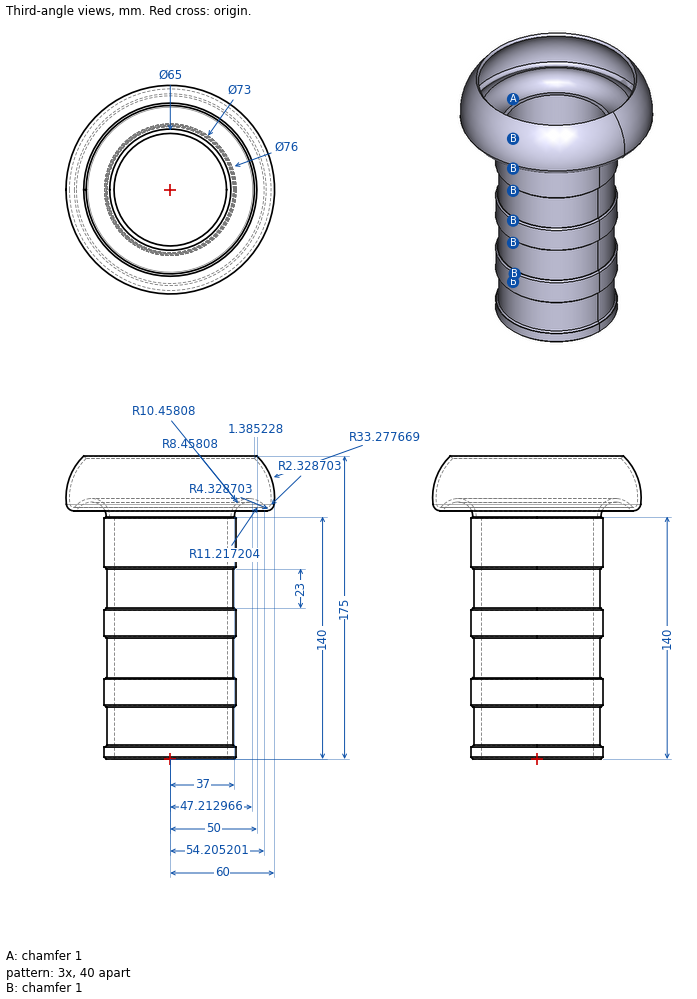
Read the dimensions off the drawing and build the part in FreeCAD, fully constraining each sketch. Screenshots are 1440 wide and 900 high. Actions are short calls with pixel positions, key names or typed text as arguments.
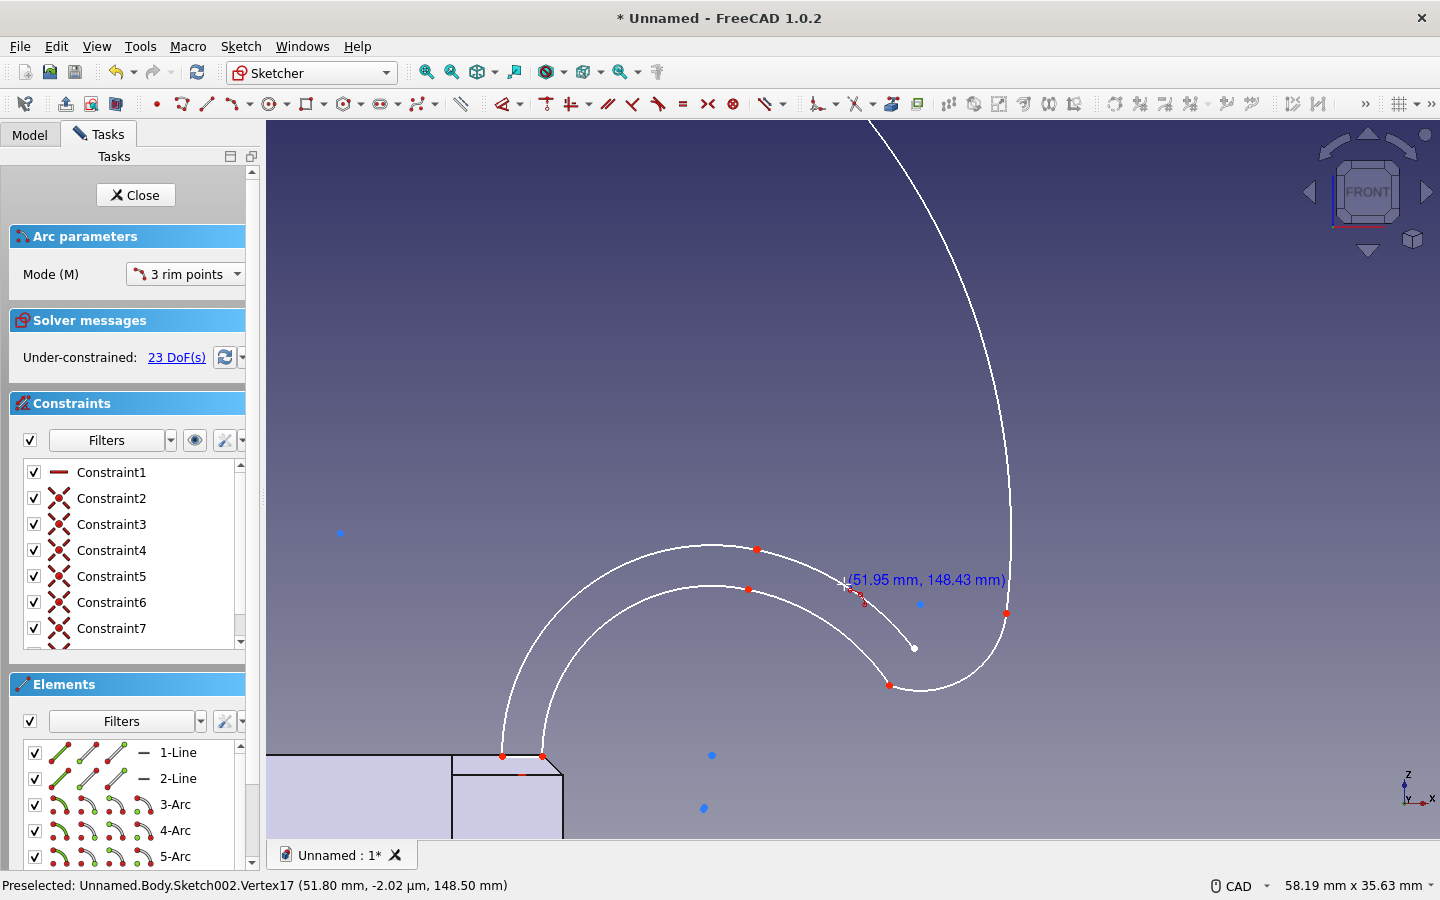
click(914, 649)
click(966, 607)
click(949, 639)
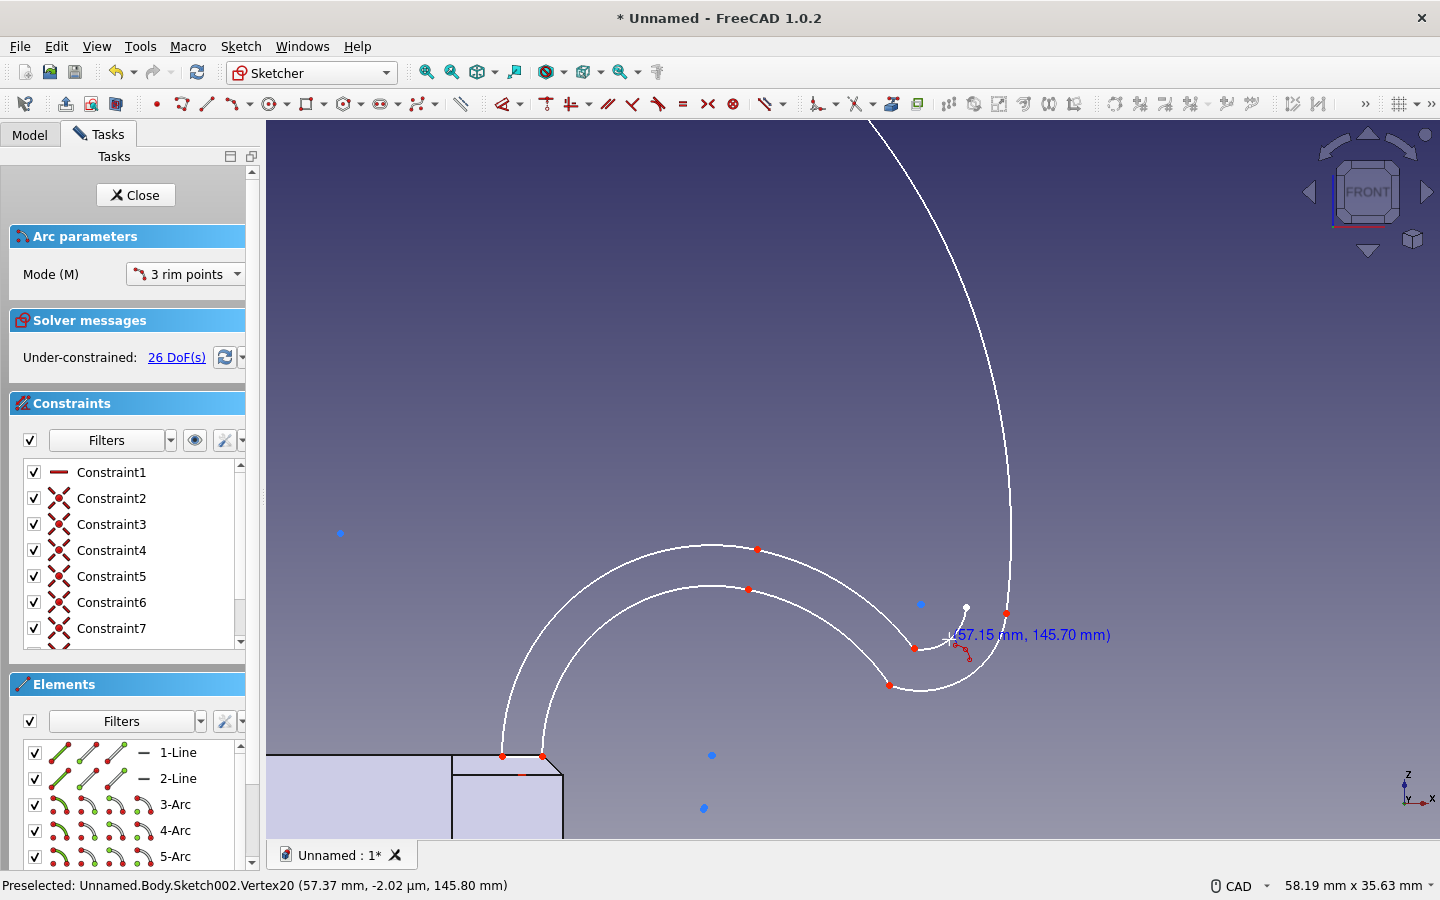
click(966, 608)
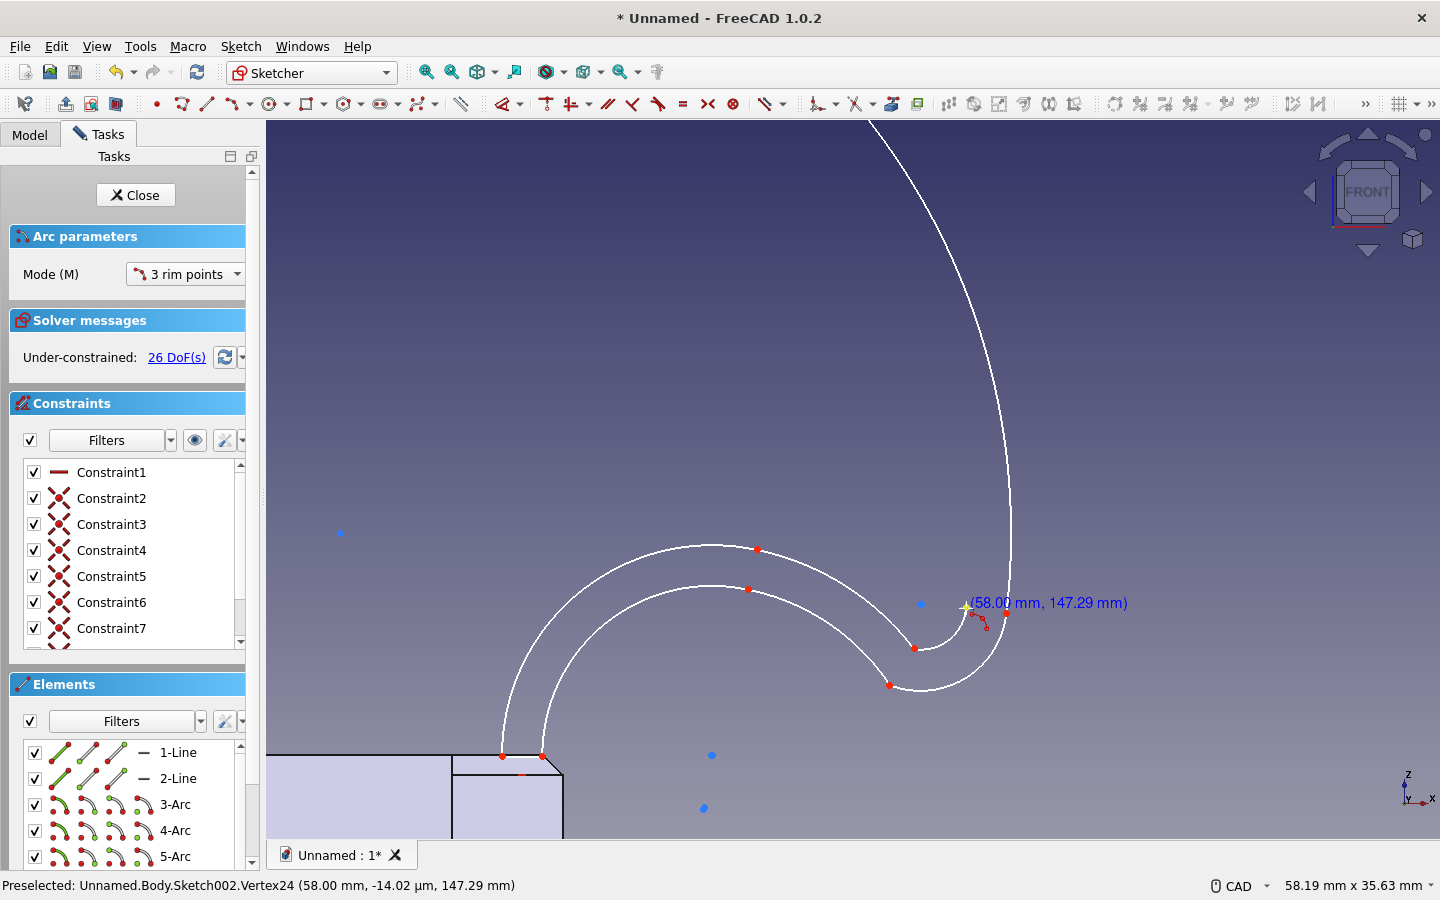
scroll(846, 637, down, 2)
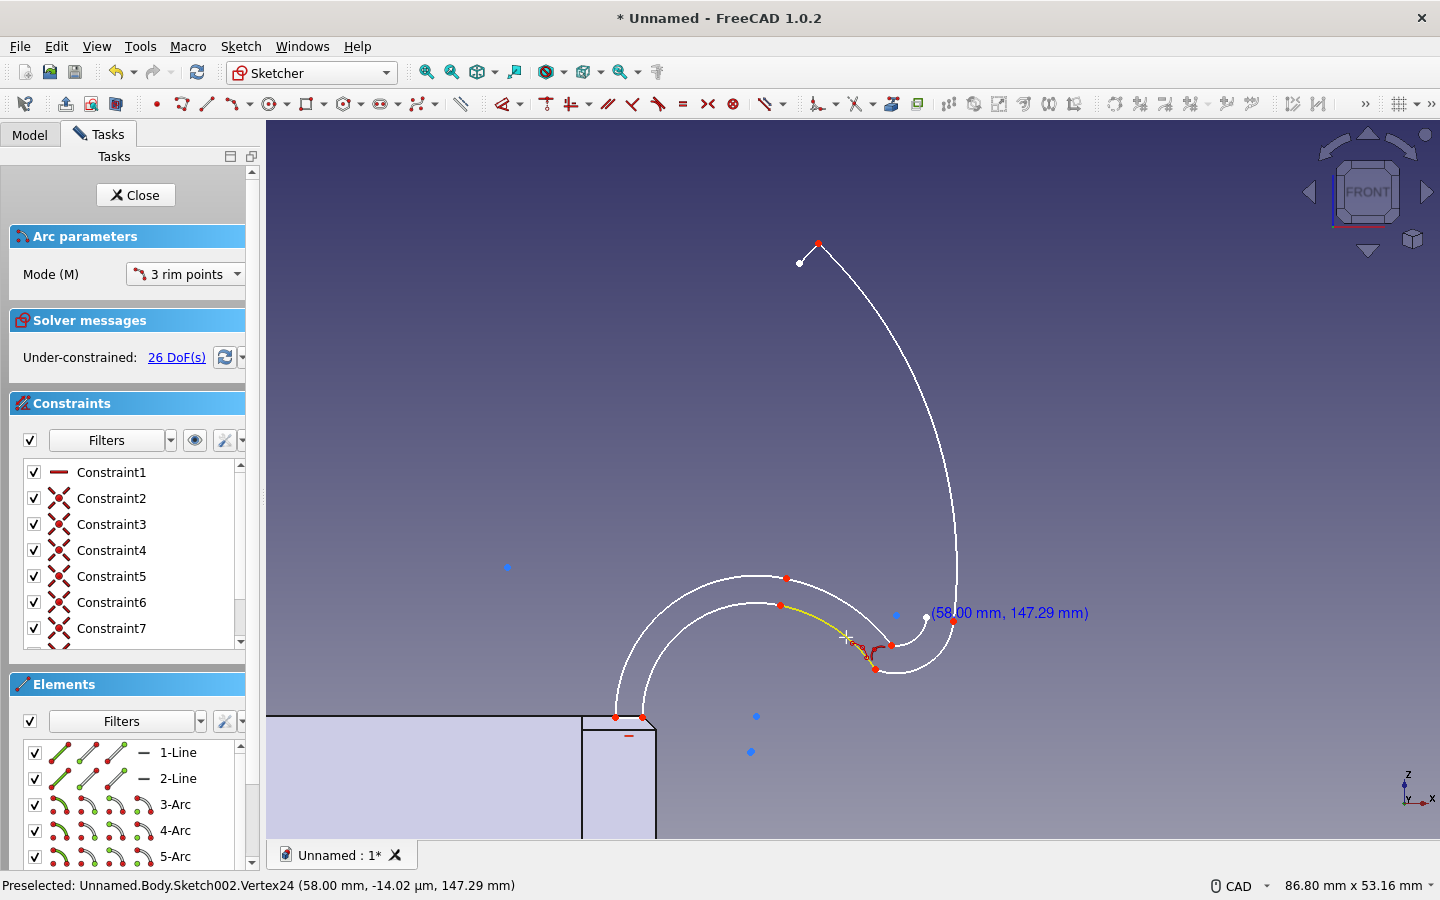
click(800, 264)
click(905, 425)
key(Escape)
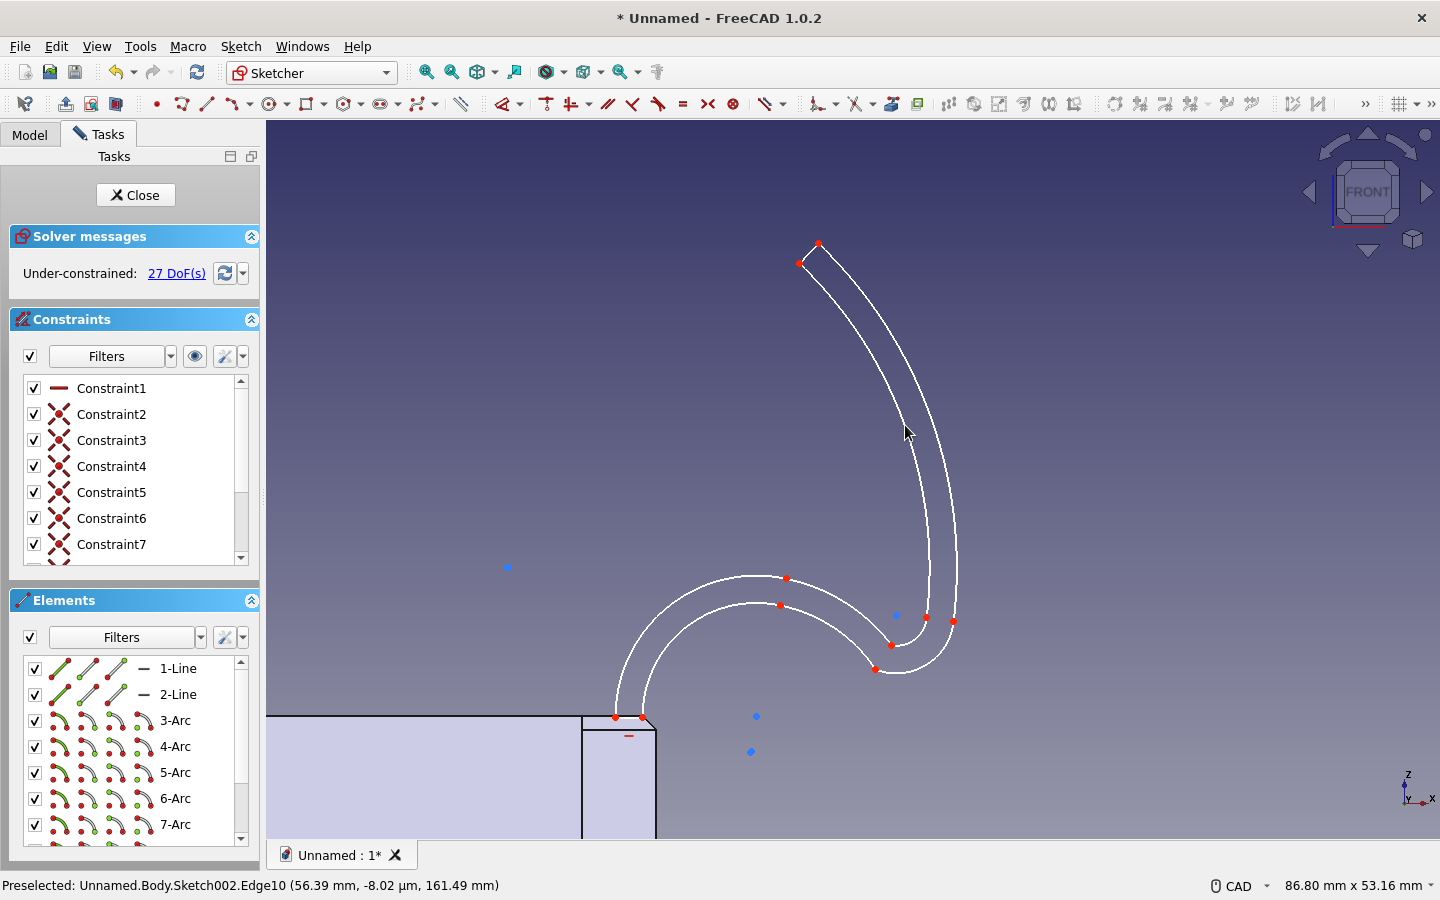
click(951, 497)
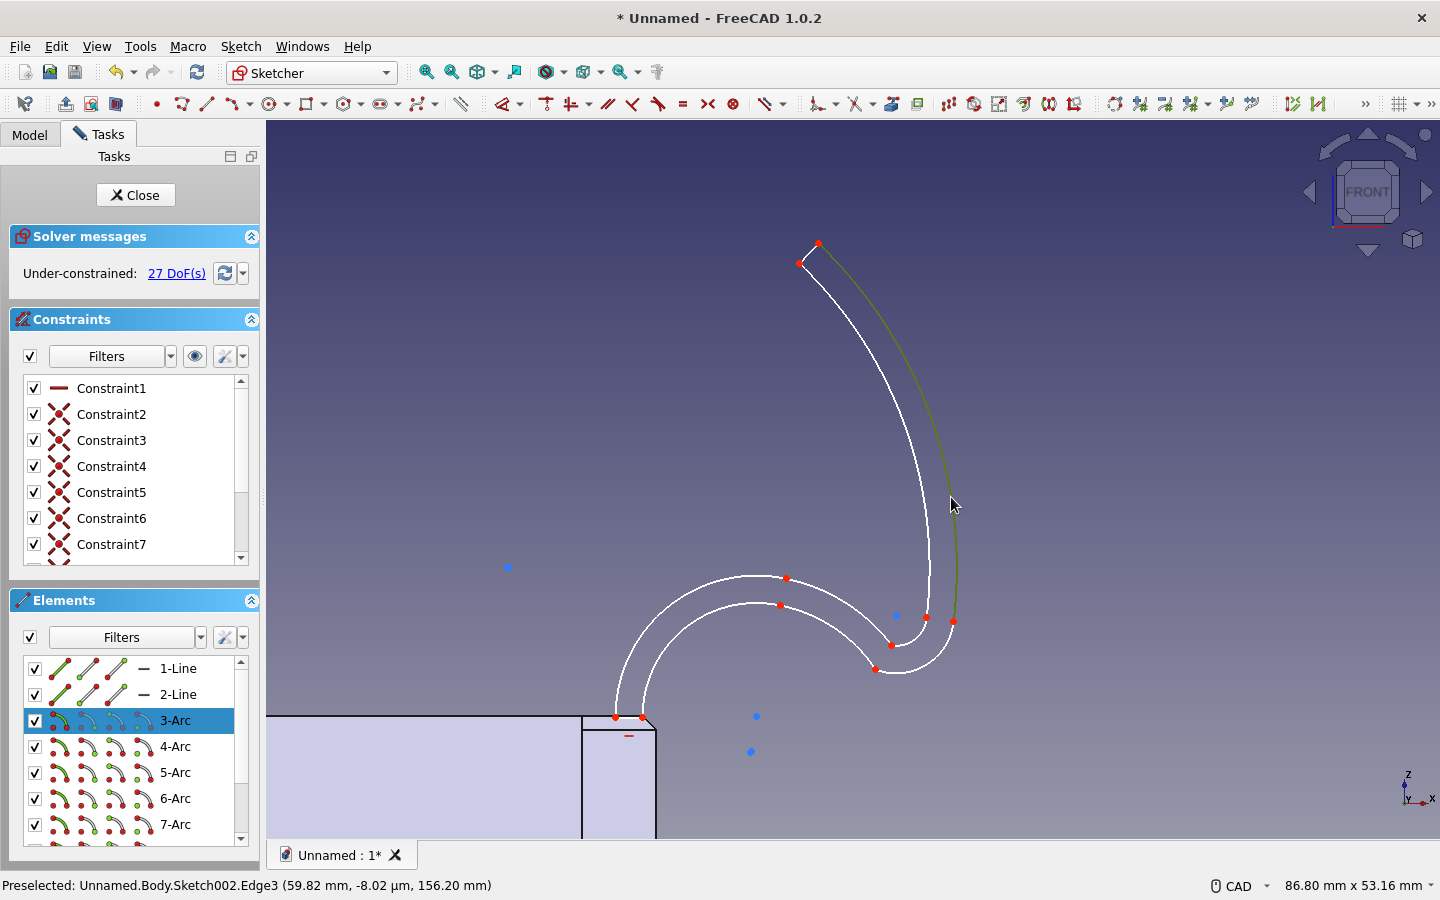
click(907, 672)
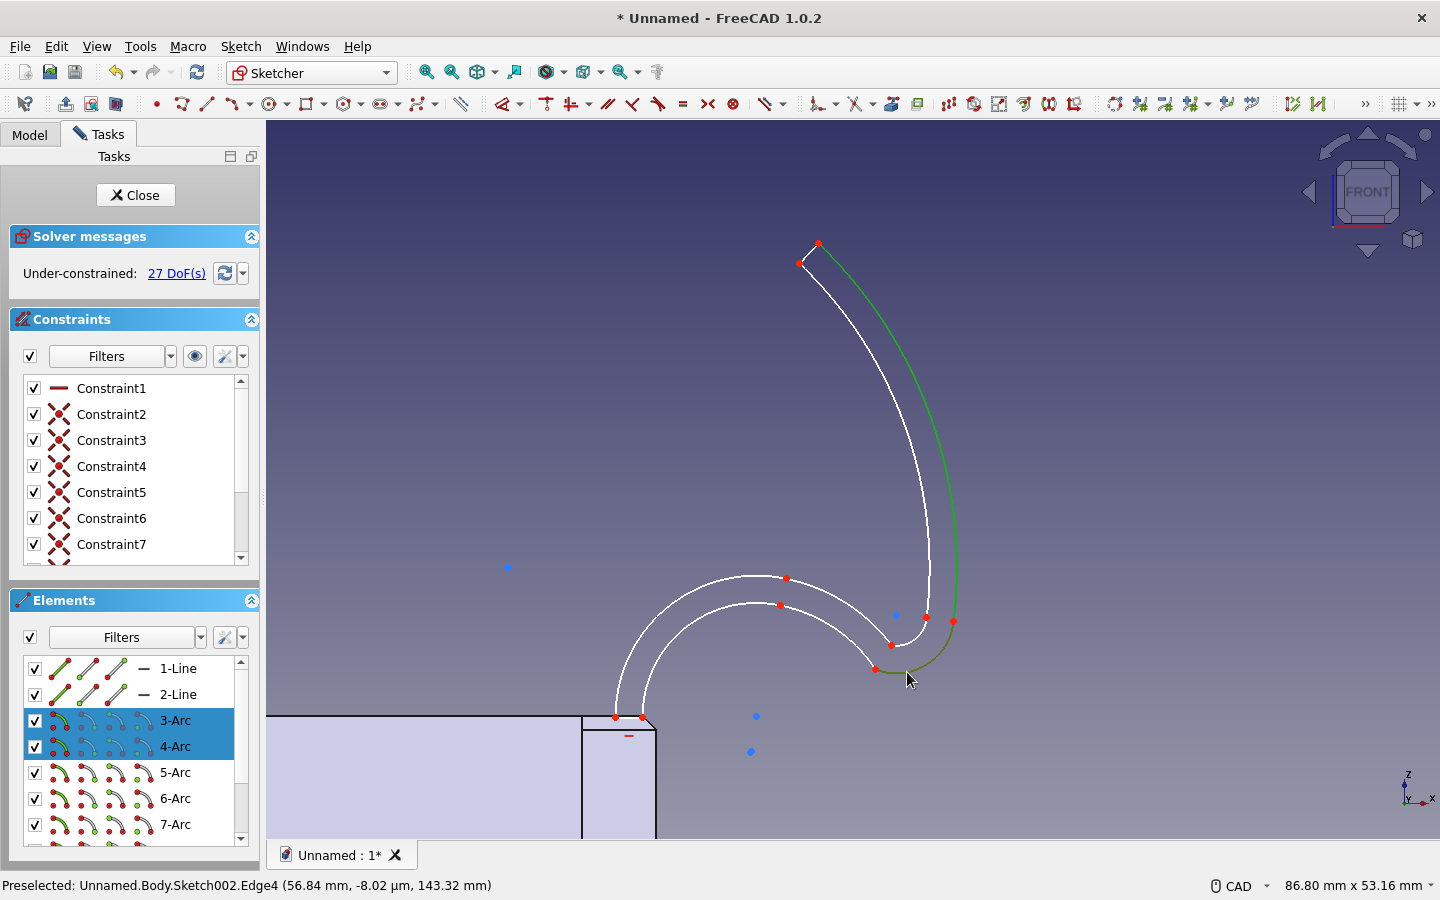
key(t)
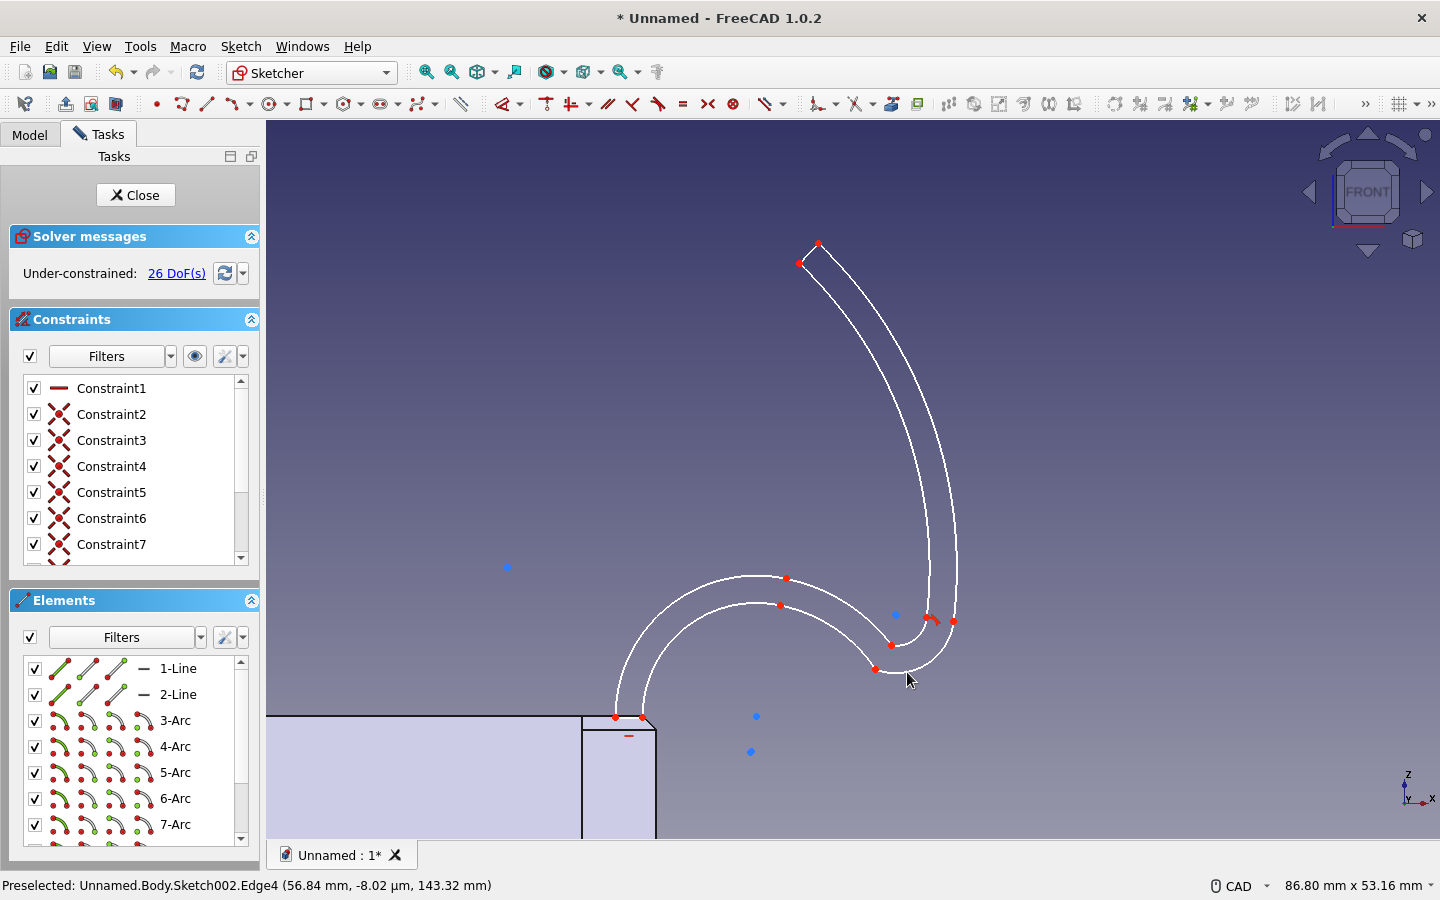
click(853, 643)